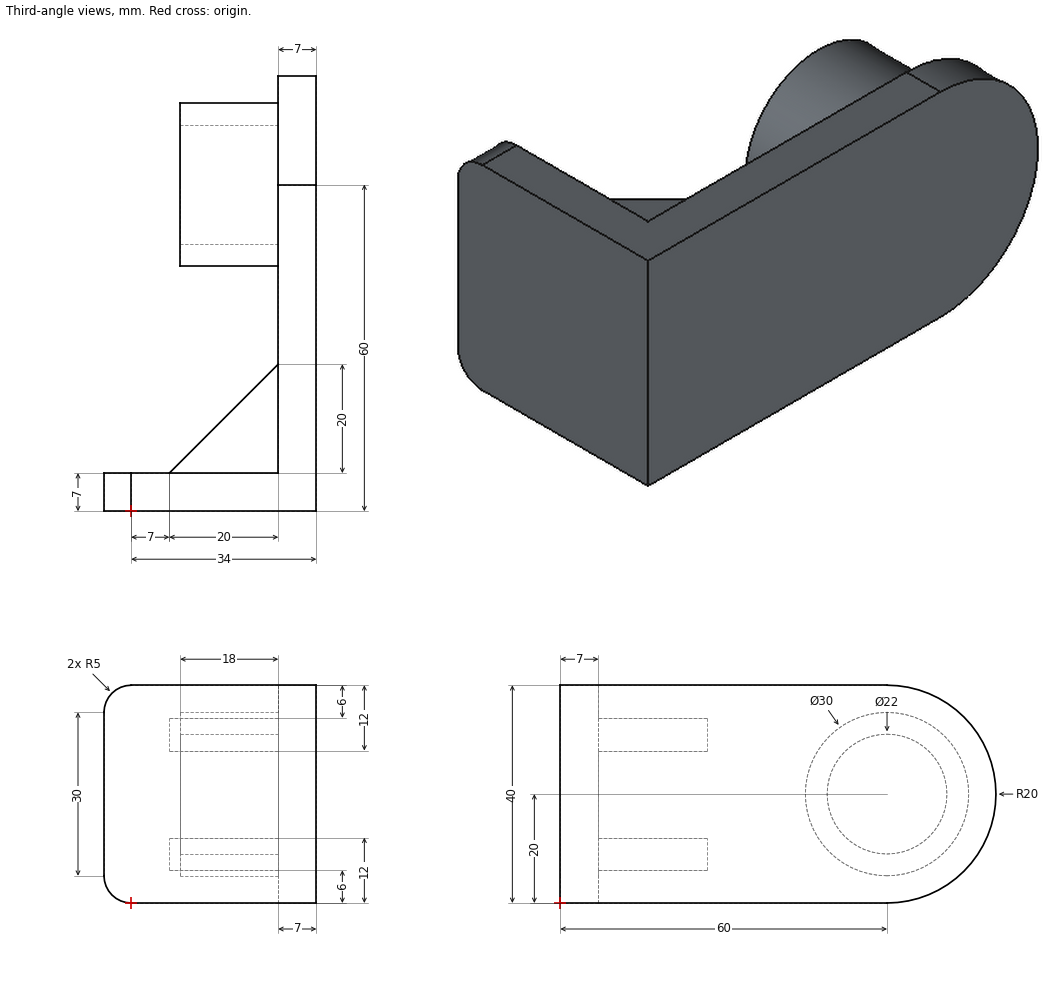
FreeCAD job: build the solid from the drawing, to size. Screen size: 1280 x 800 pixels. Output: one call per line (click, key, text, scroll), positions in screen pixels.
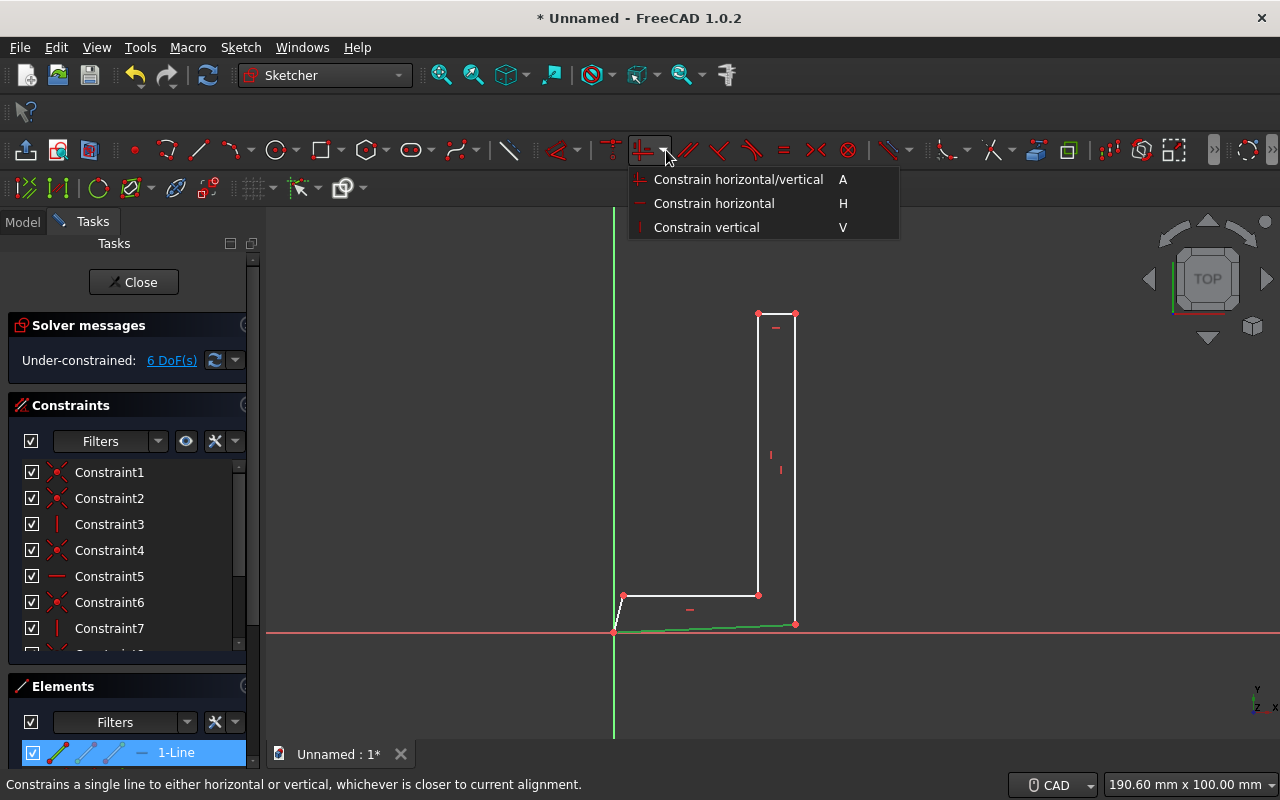
click(764, 203)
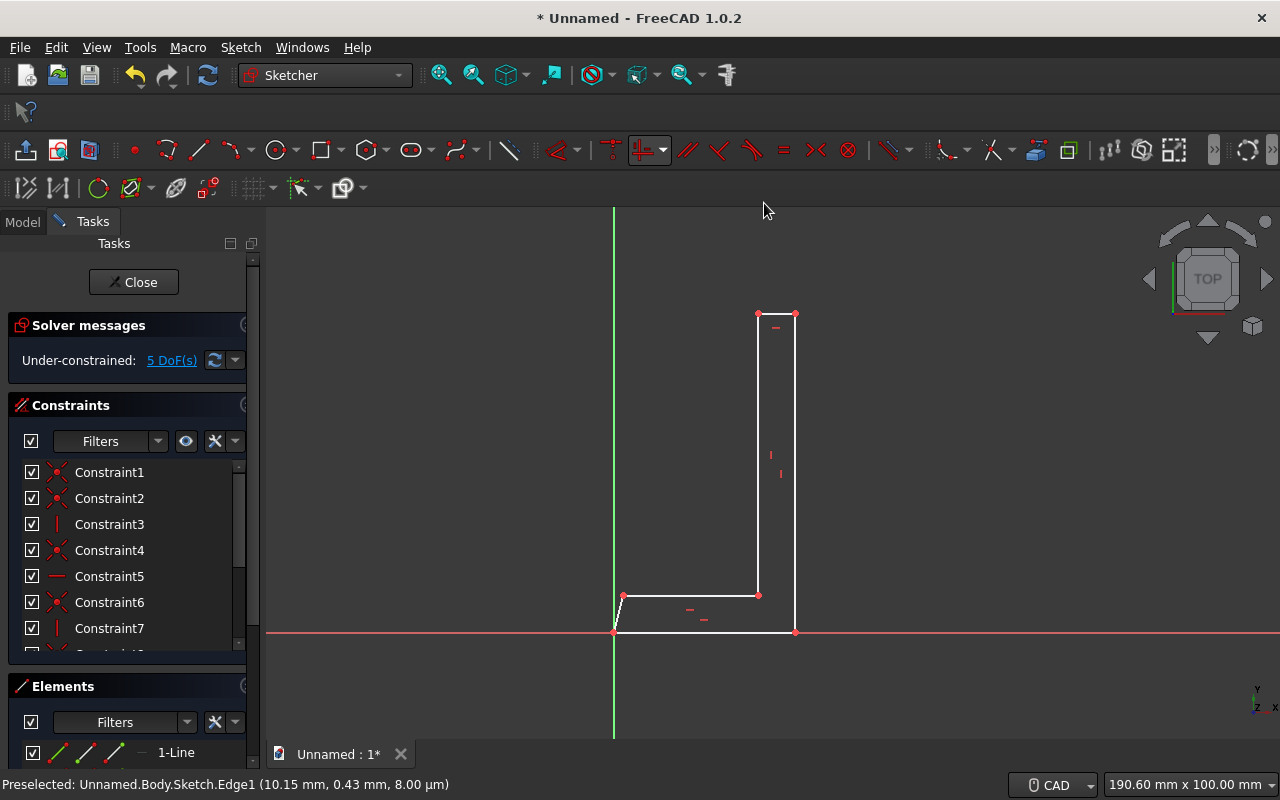
scroll(617, 622, up, 2)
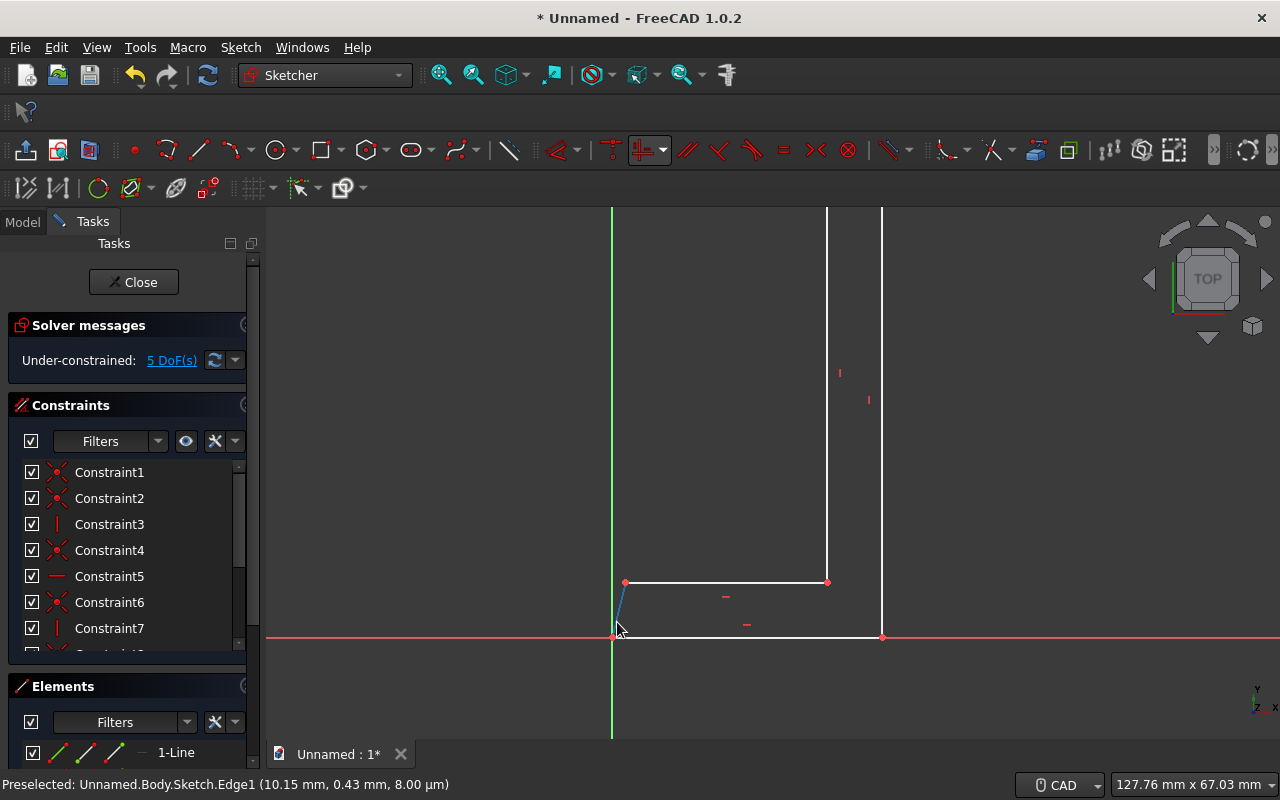
click(616, 621)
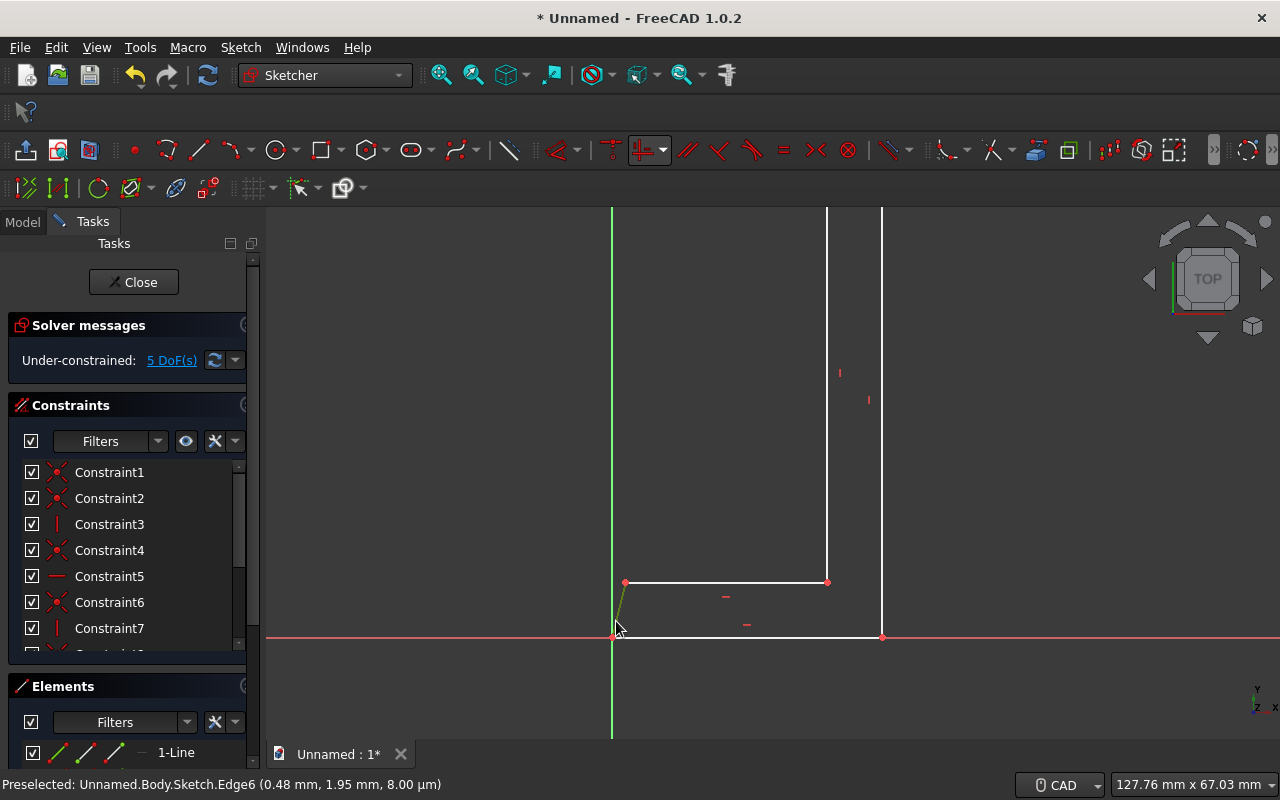
key(v)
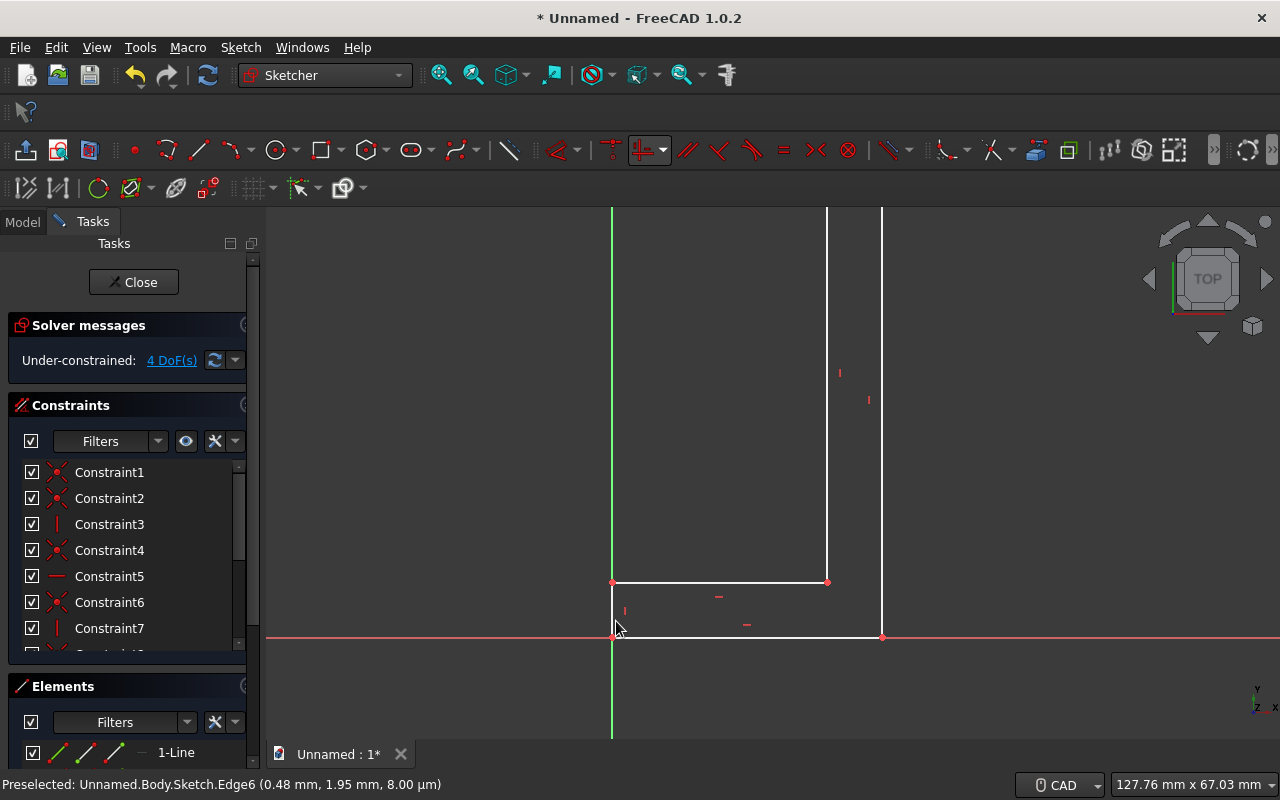
click(556, 150)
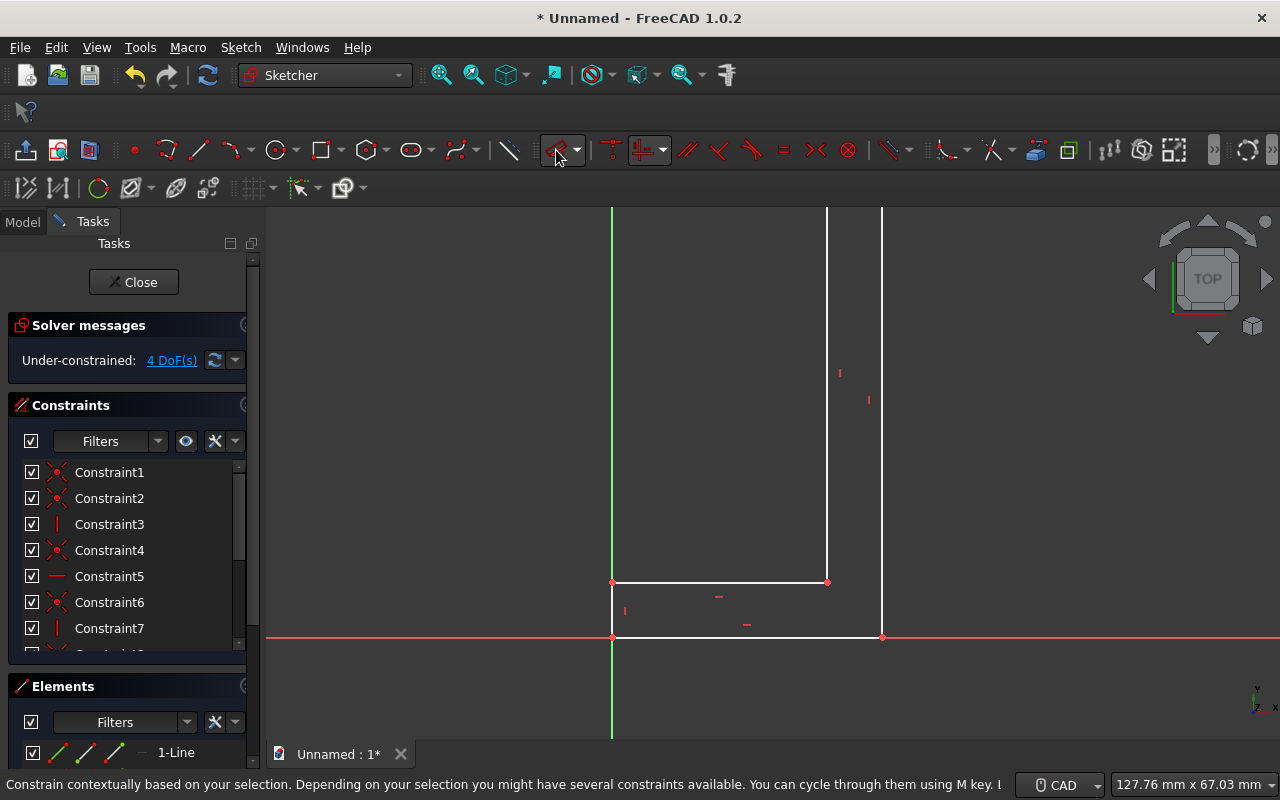
scroll(618, 623, down, 2)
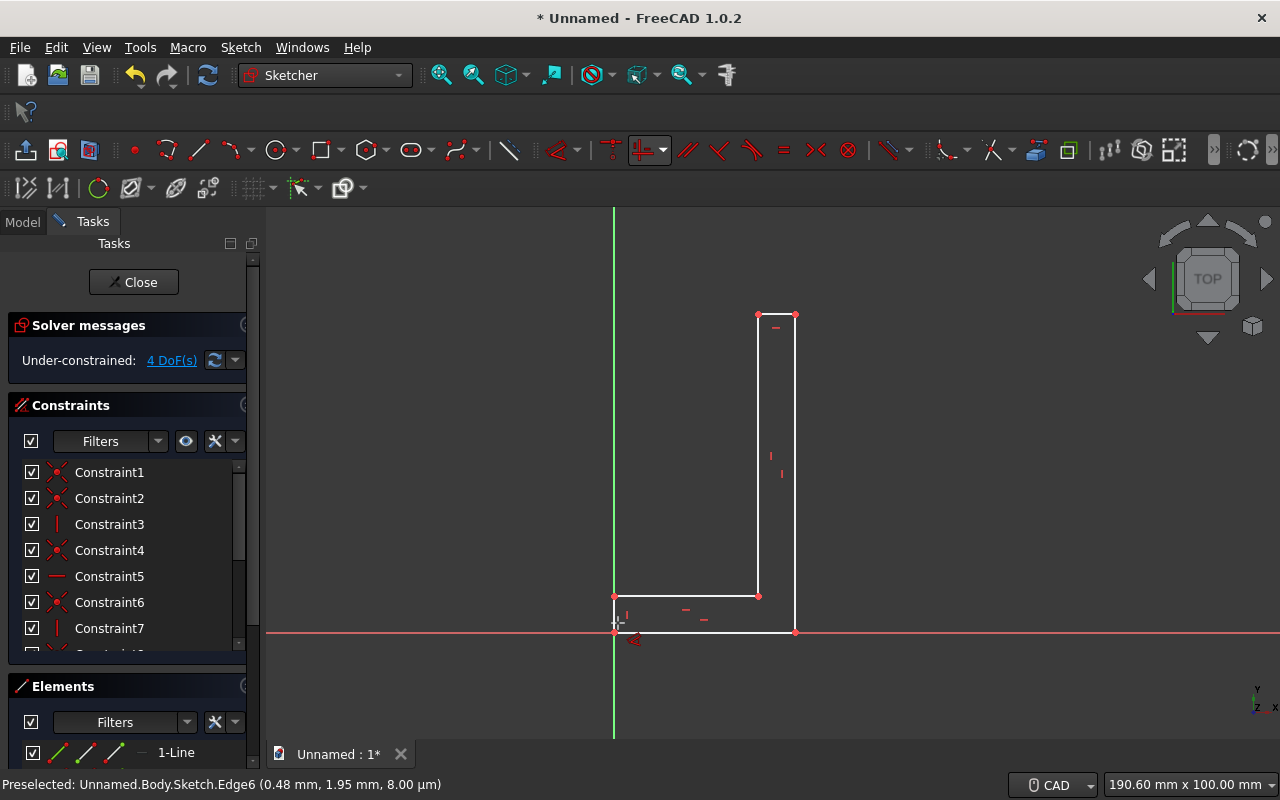
scroll(784, 314, up, 2)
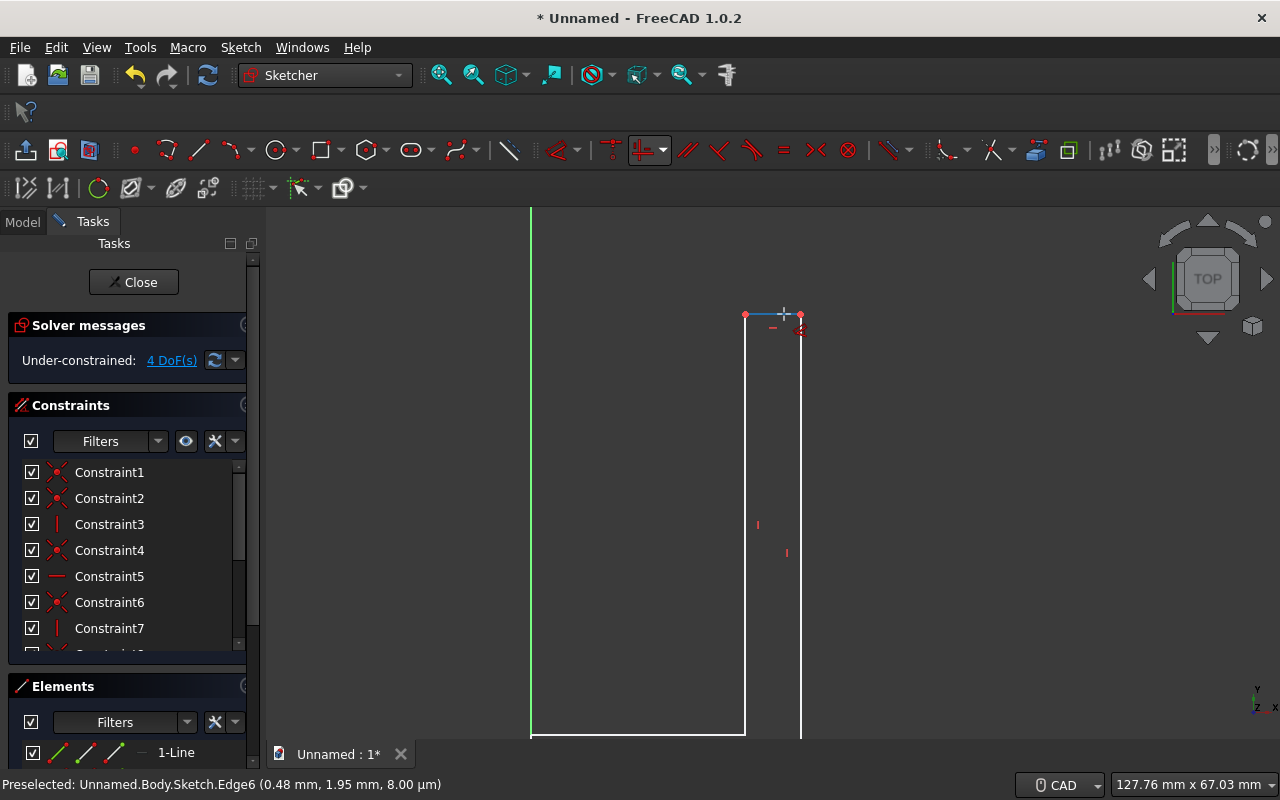
click(784, 314)
click(773, 280)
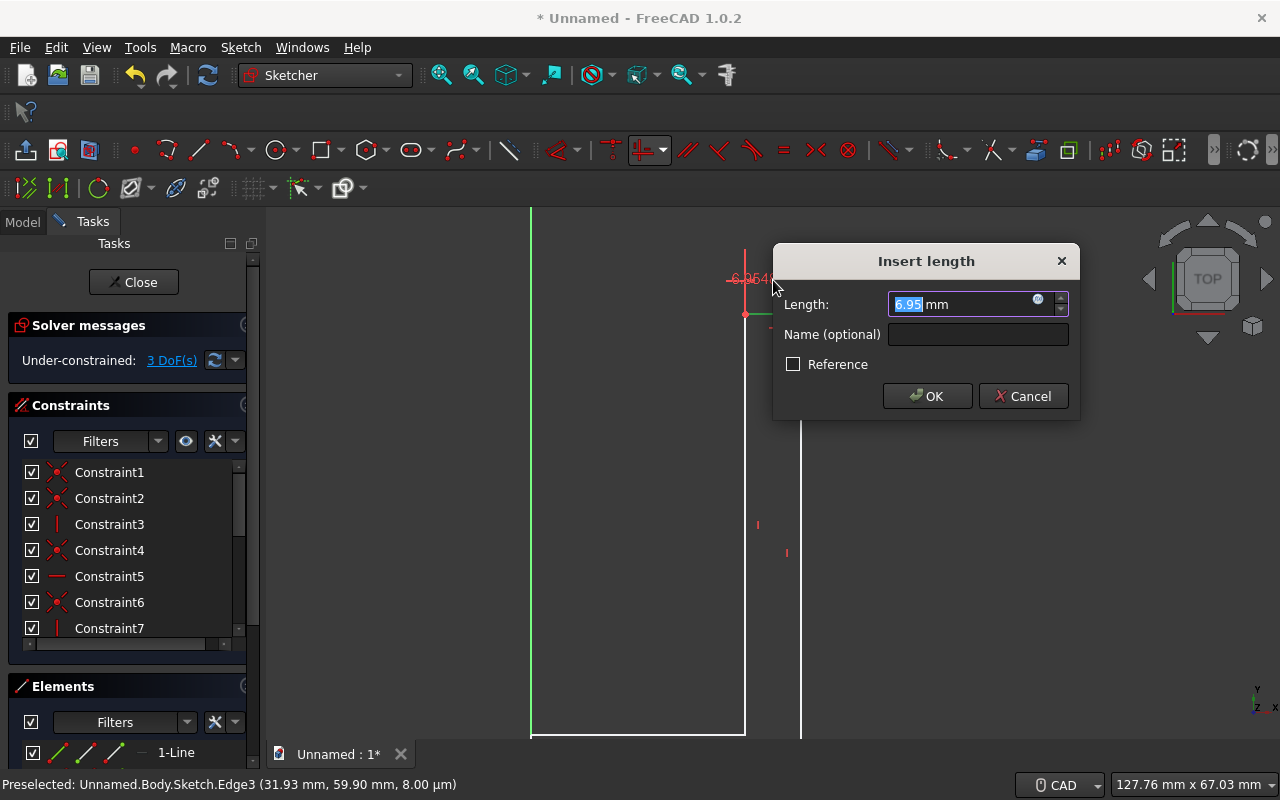
text(7)
key(Return)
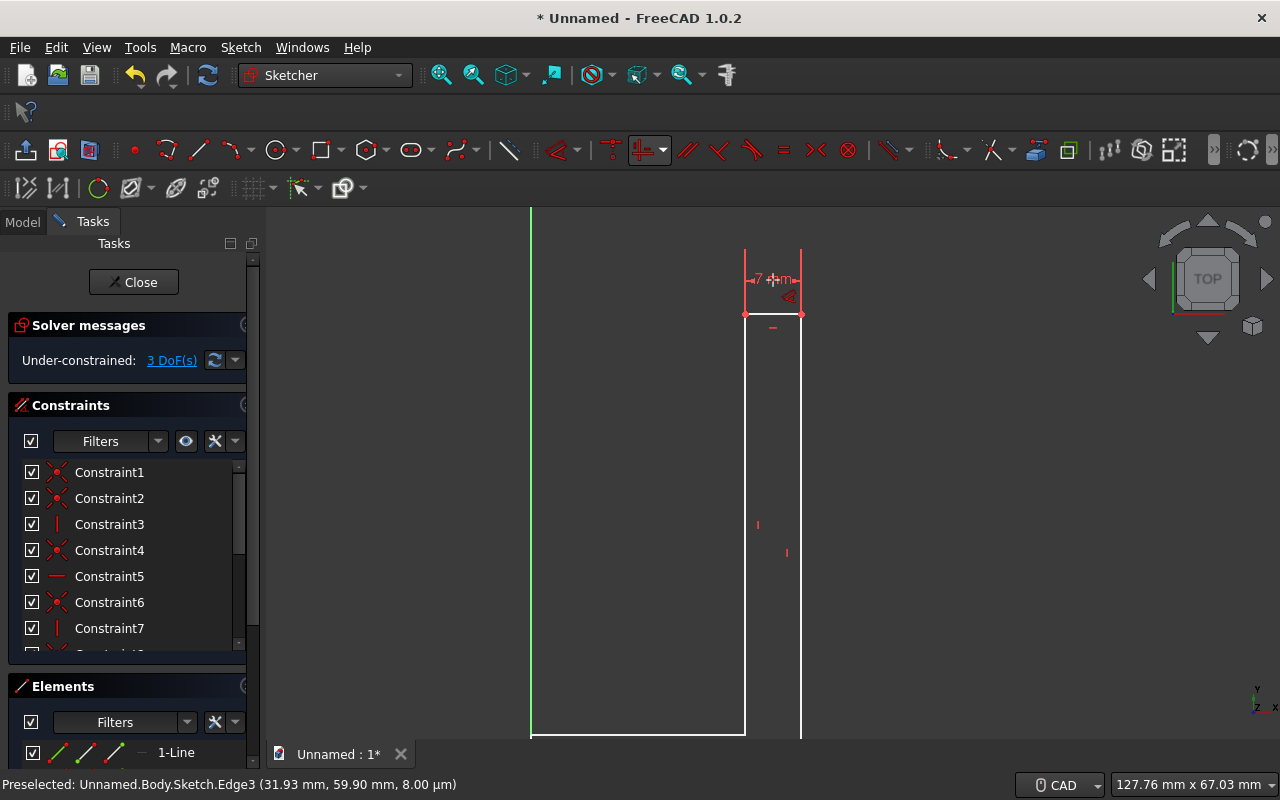
scroll(784, 313, down, 2)